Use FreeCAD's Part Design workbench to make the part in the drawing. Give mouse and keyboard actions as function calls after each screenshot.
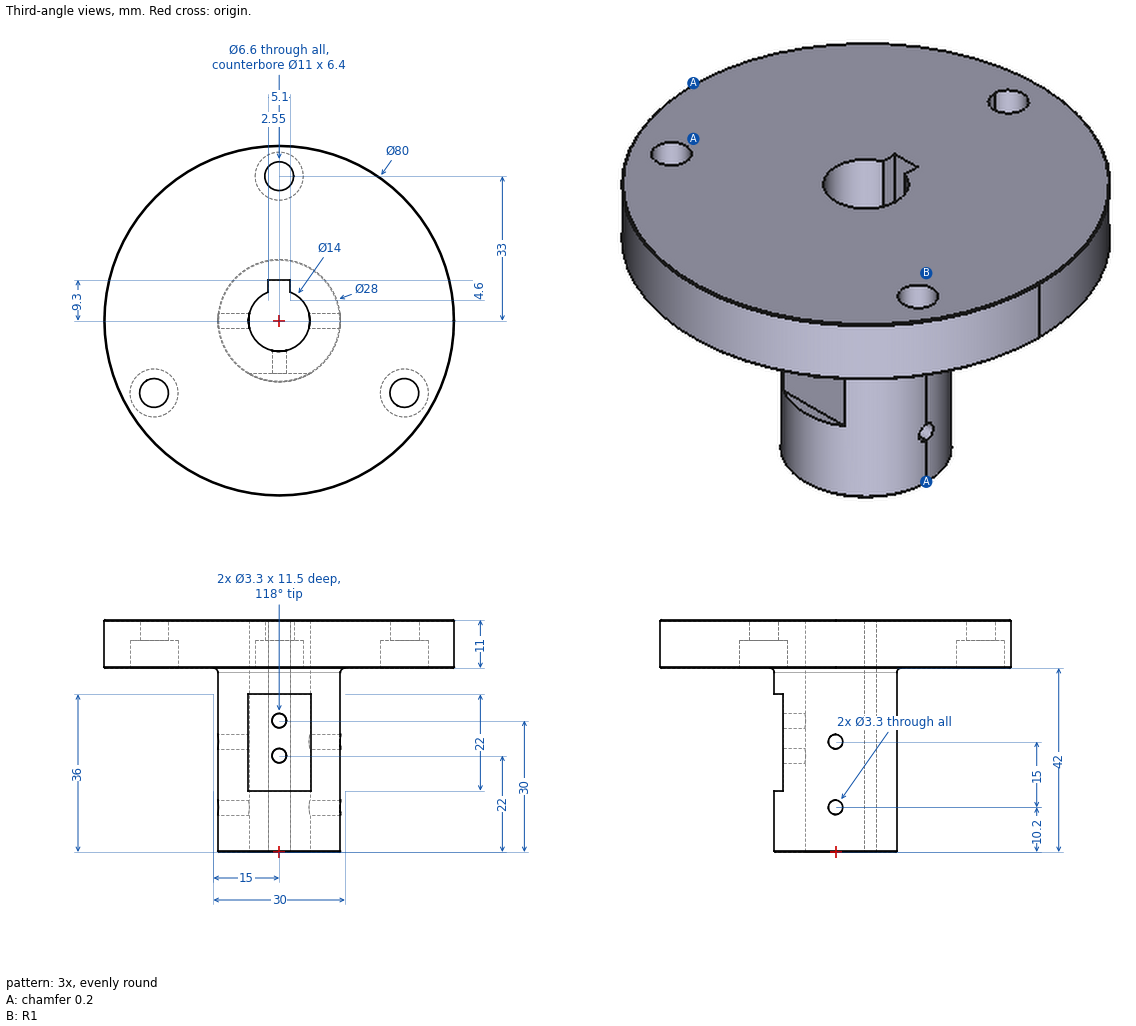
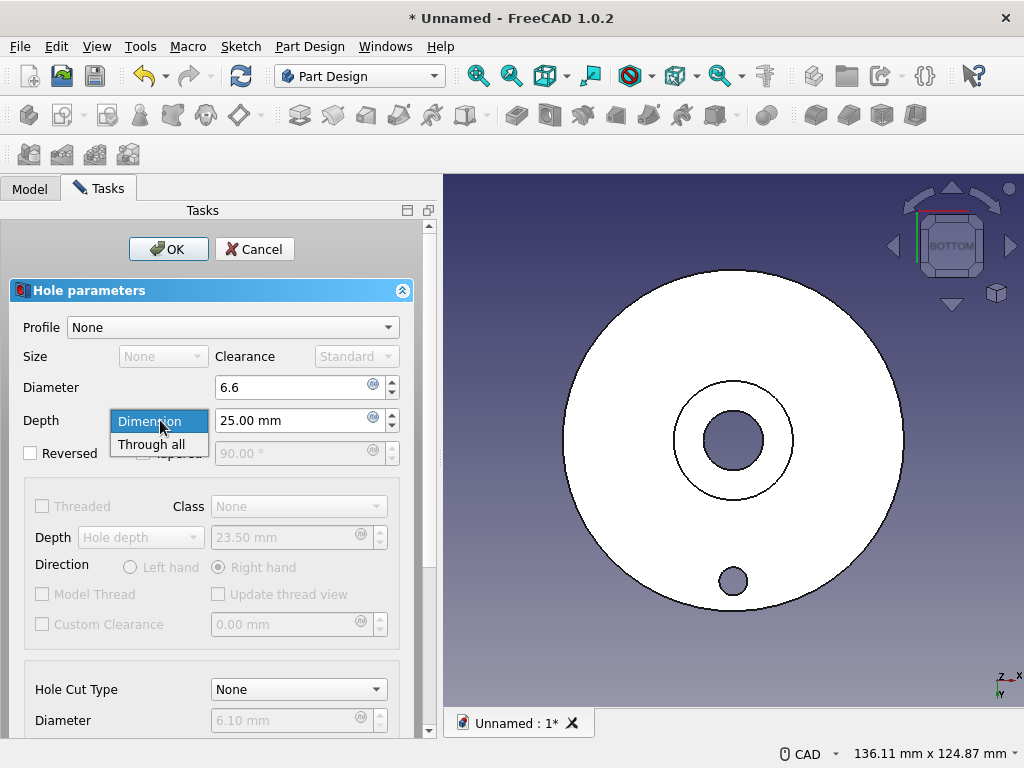
click(158, 444)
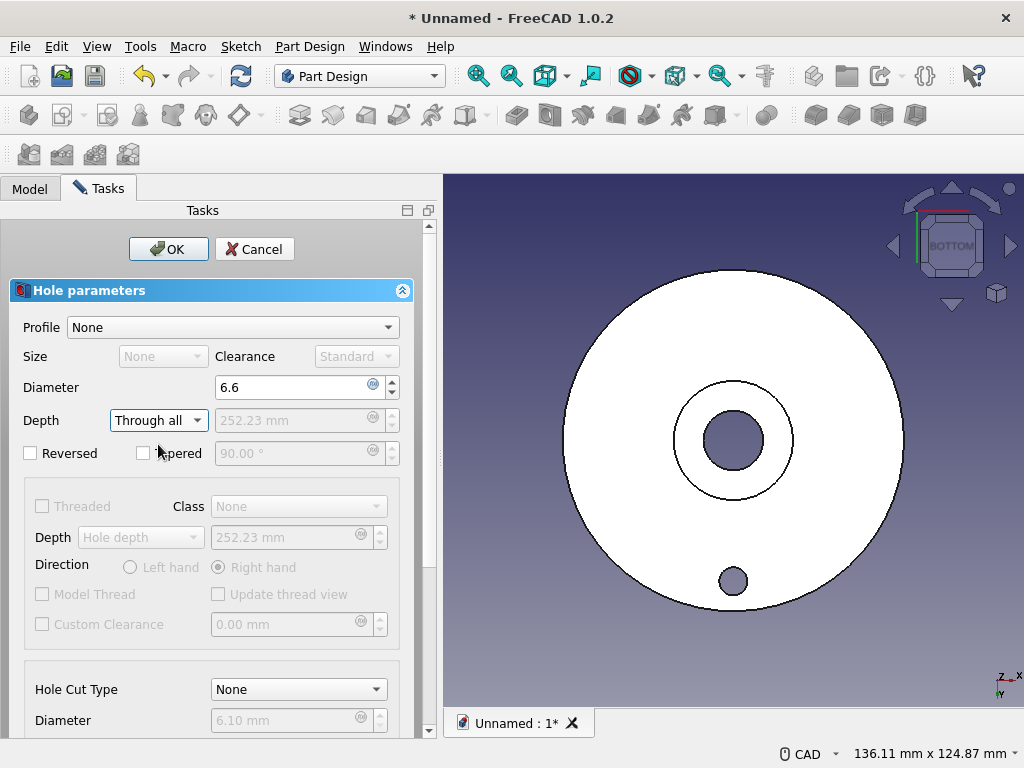
click(300, 690)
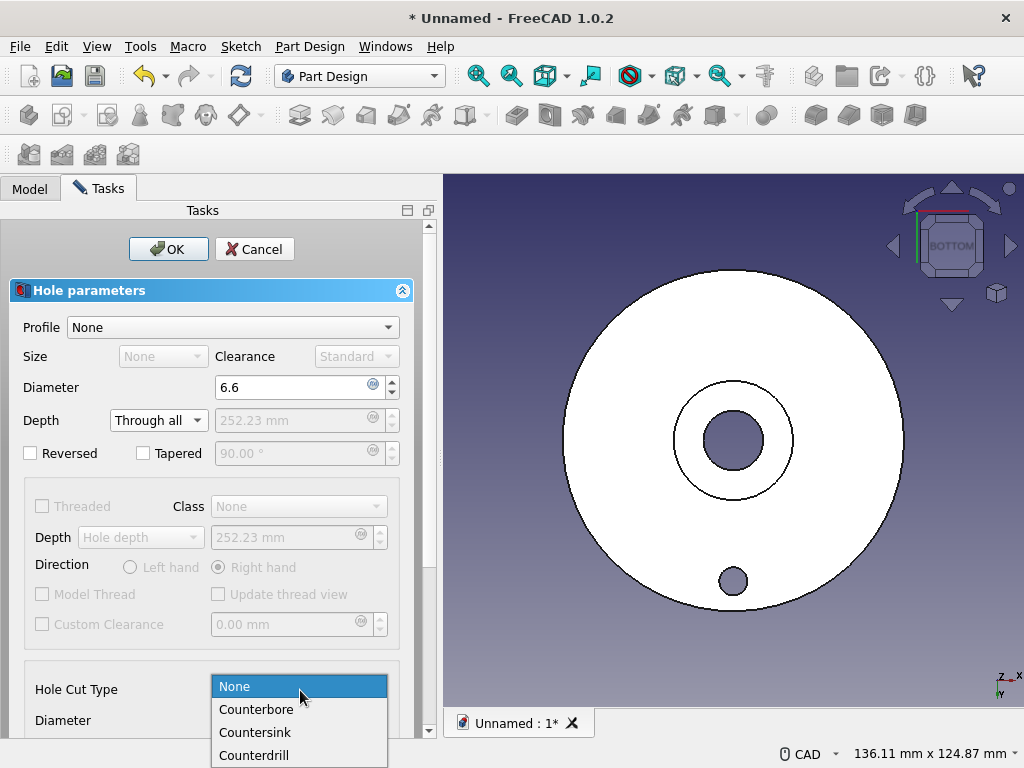
click(298, 710)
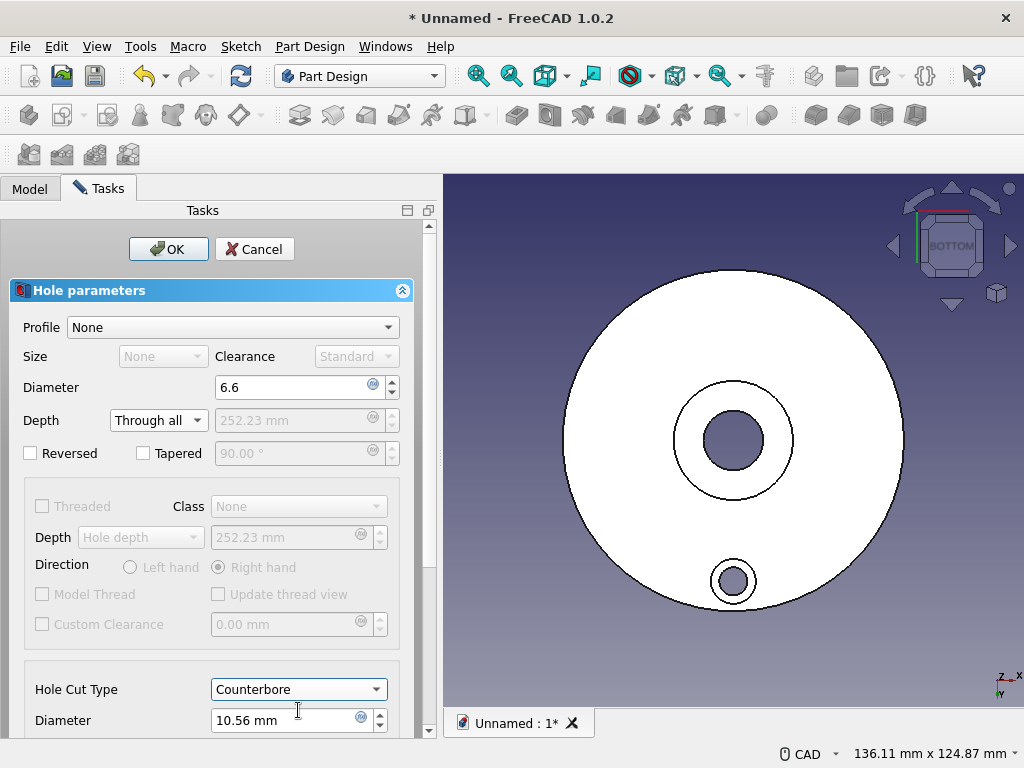
triple_click(292, 720)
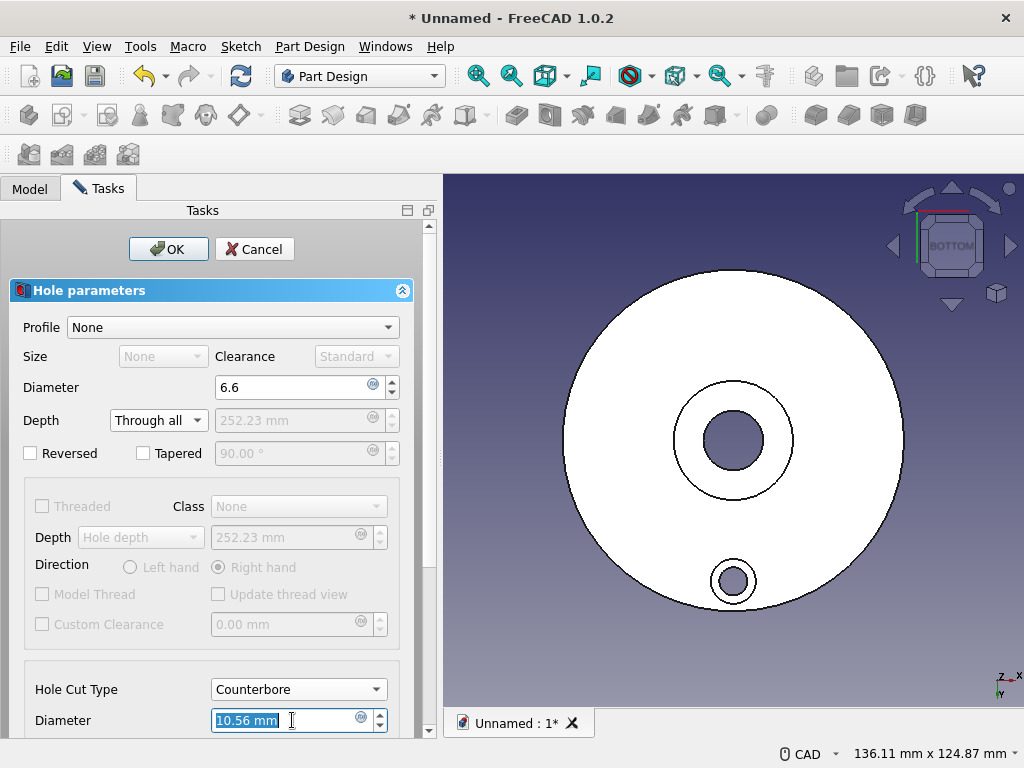
text(11)
key(Tab)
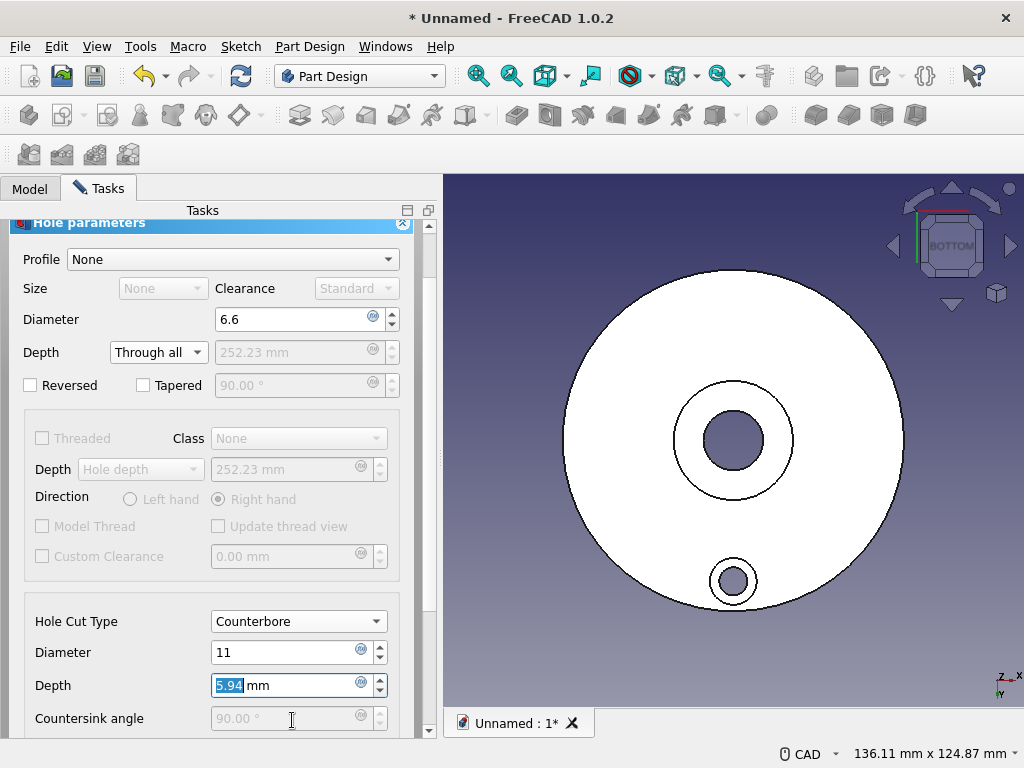
text(6.4)
key(Tab)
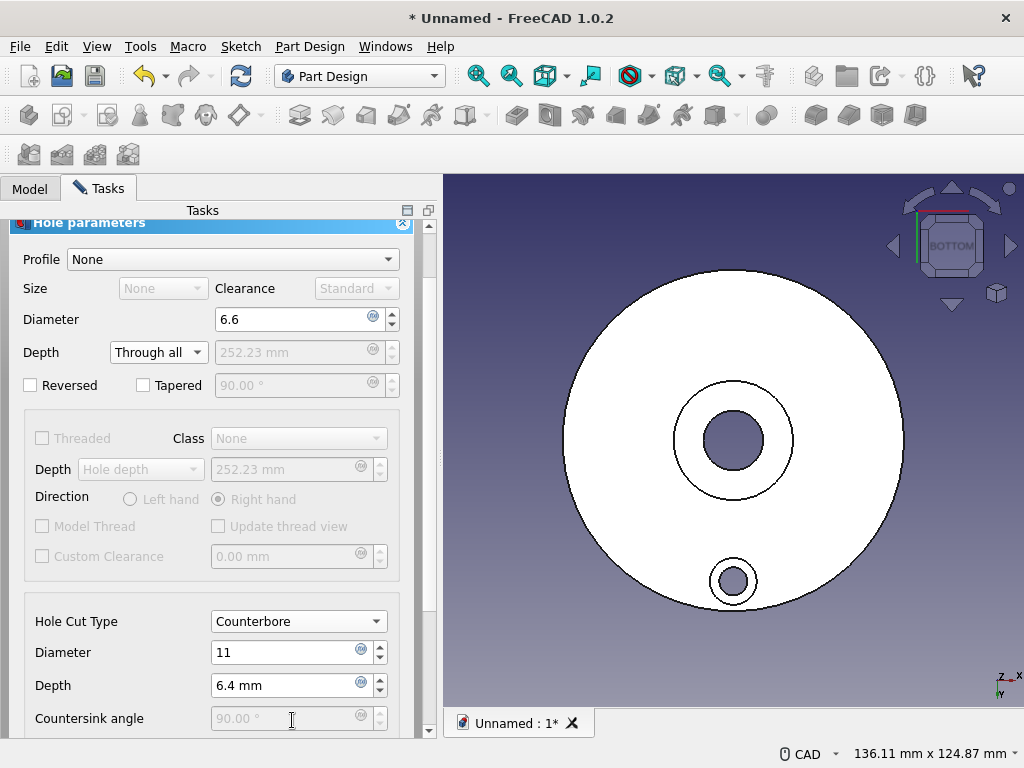
scroll(429, 479, up, 2)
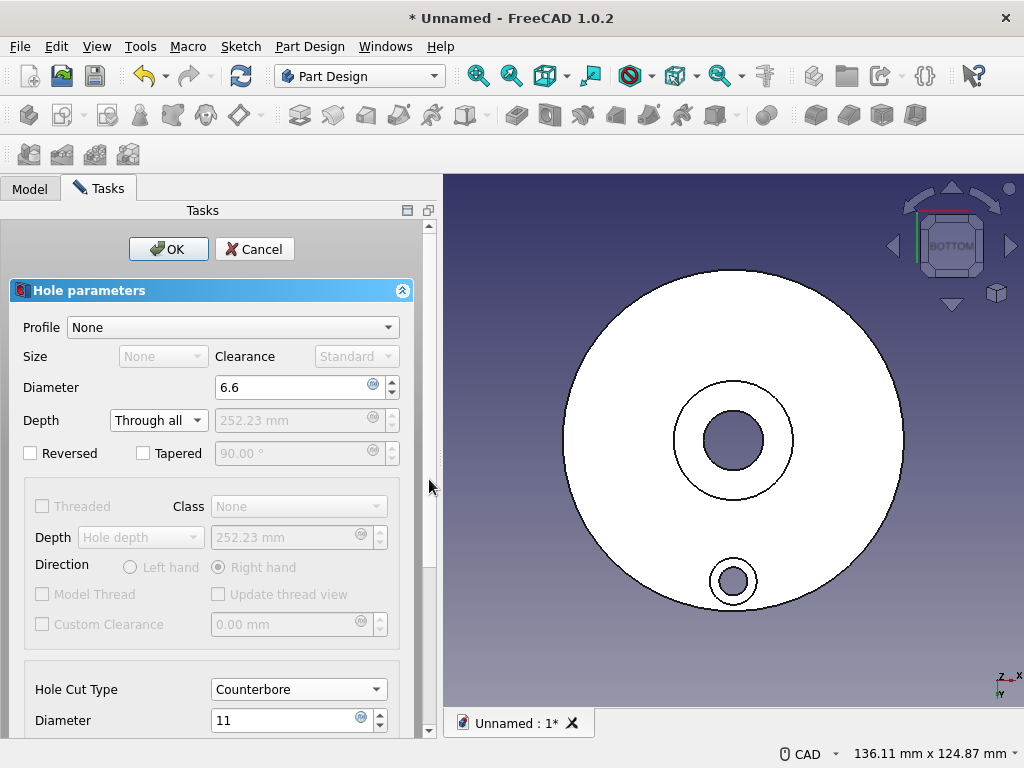
click(169, 249)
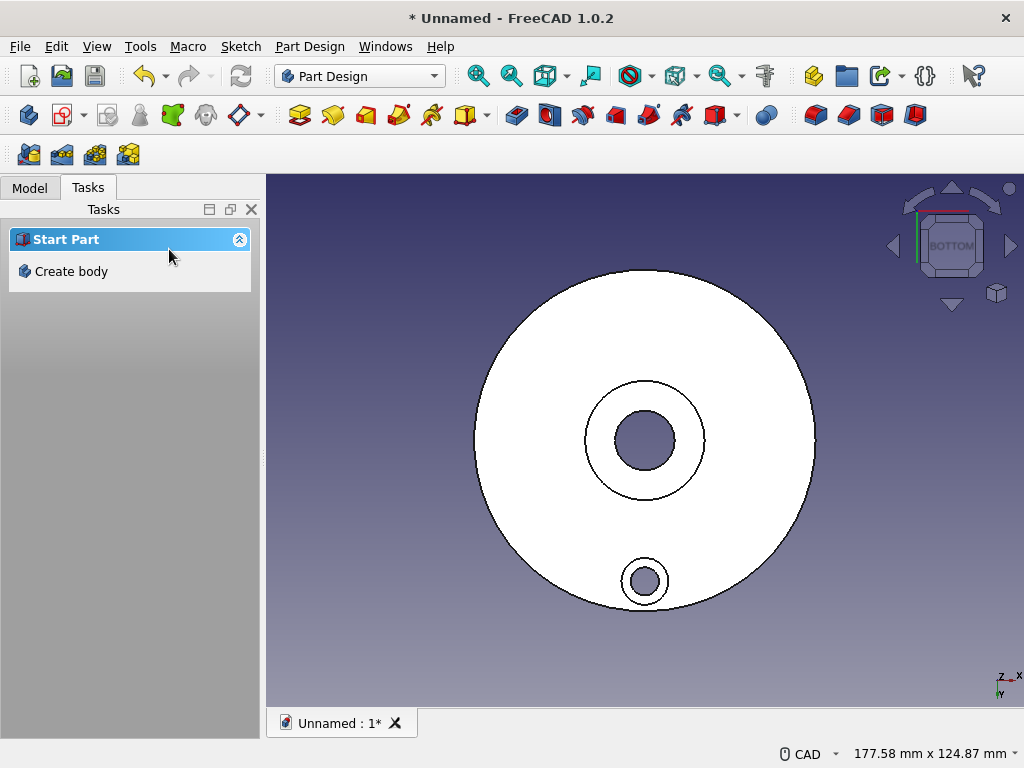
click(30, 188)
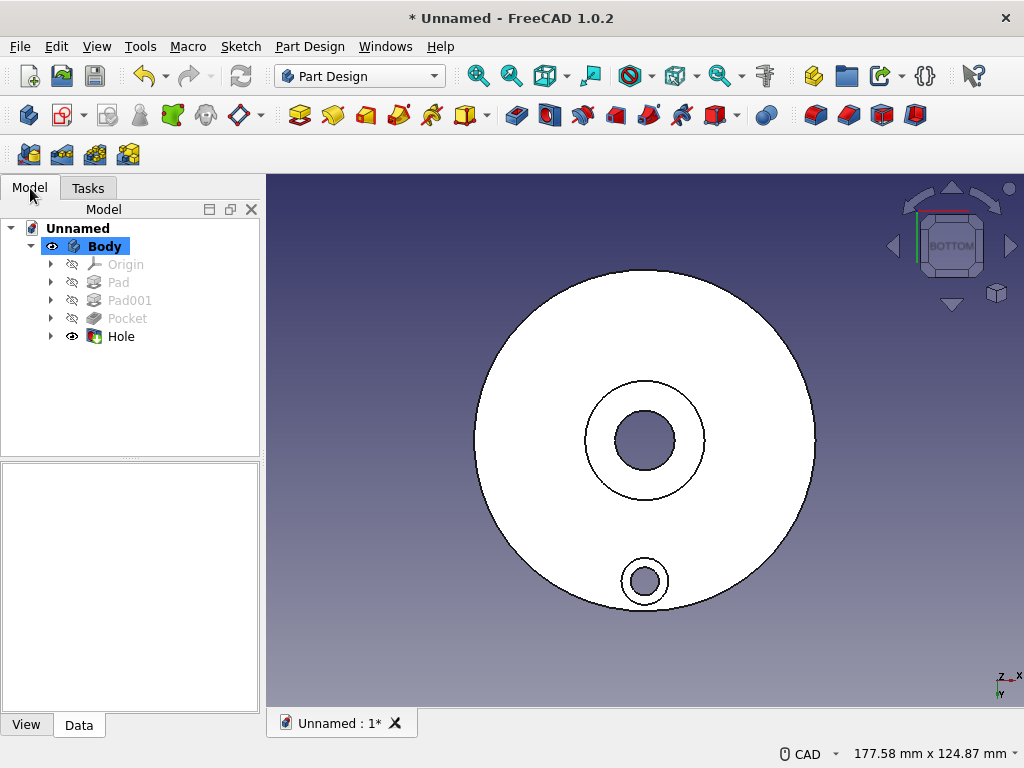
click(117, 336)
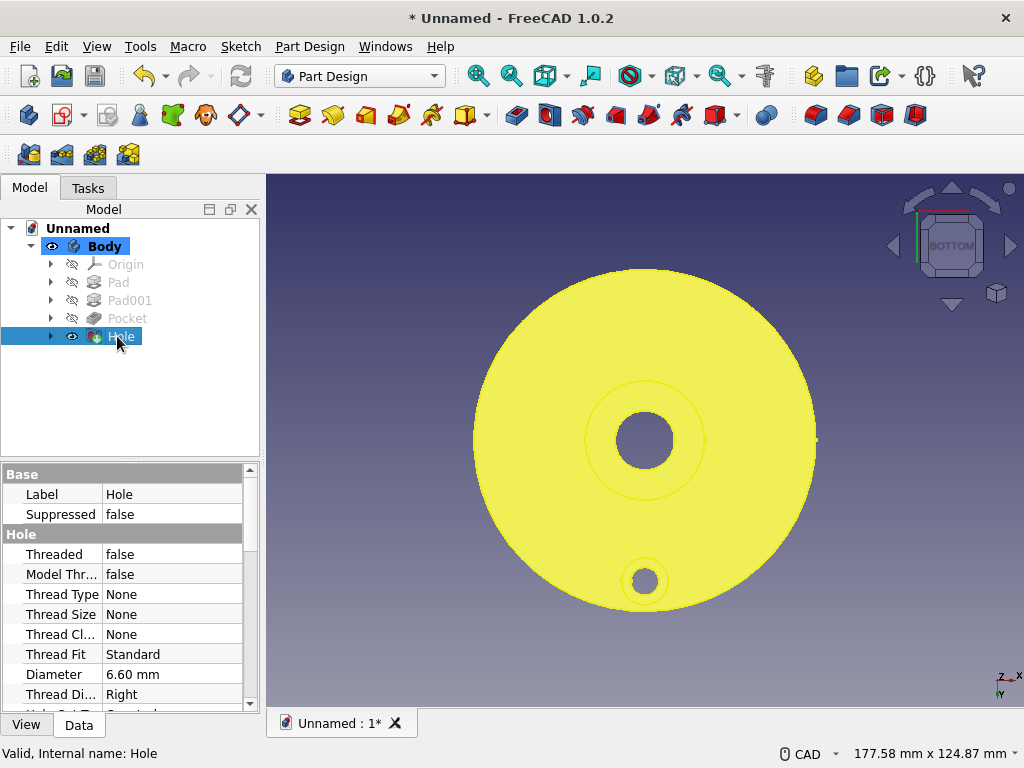
click(95, 154)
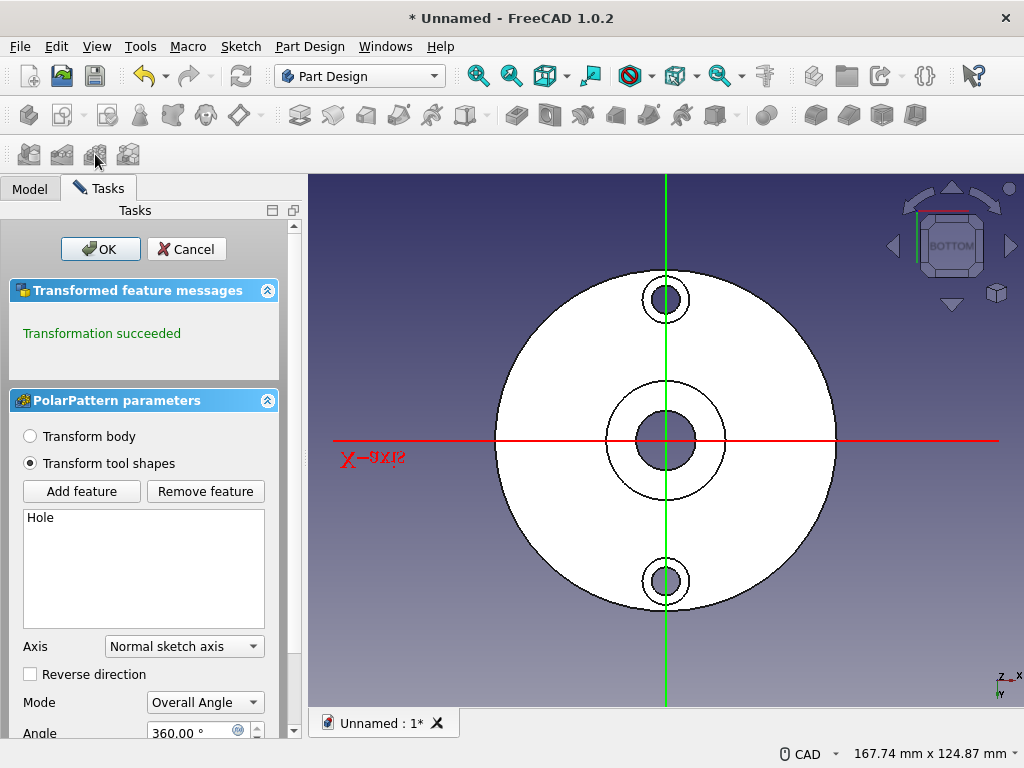
click(185, 646)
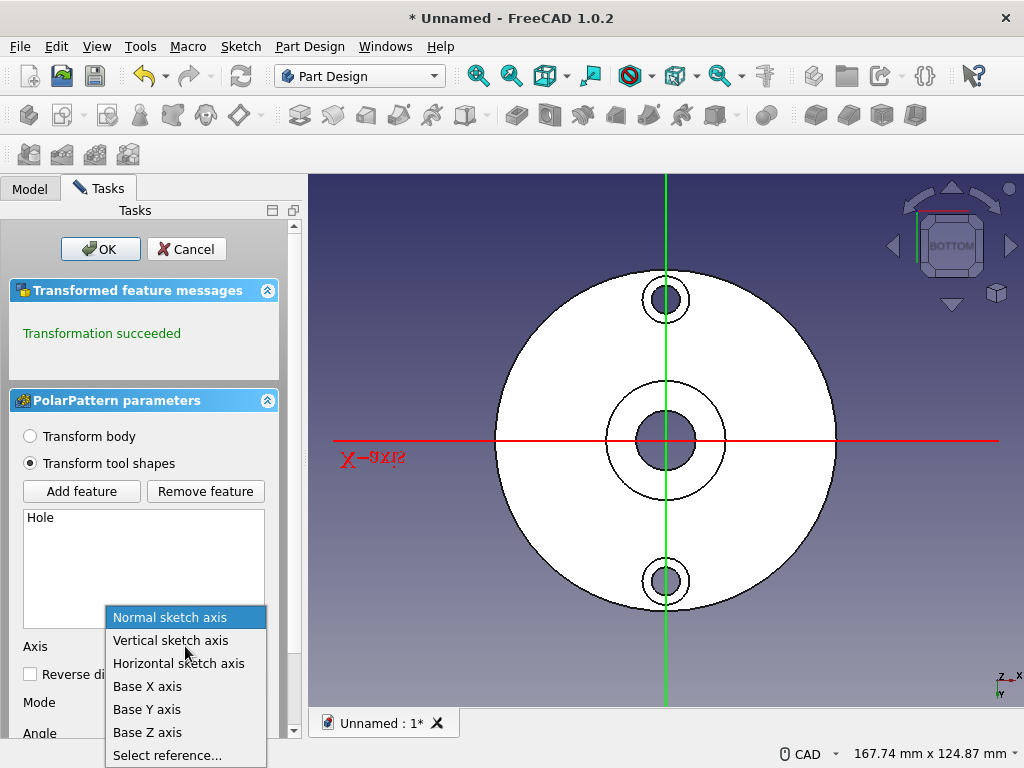
click(184, 732)